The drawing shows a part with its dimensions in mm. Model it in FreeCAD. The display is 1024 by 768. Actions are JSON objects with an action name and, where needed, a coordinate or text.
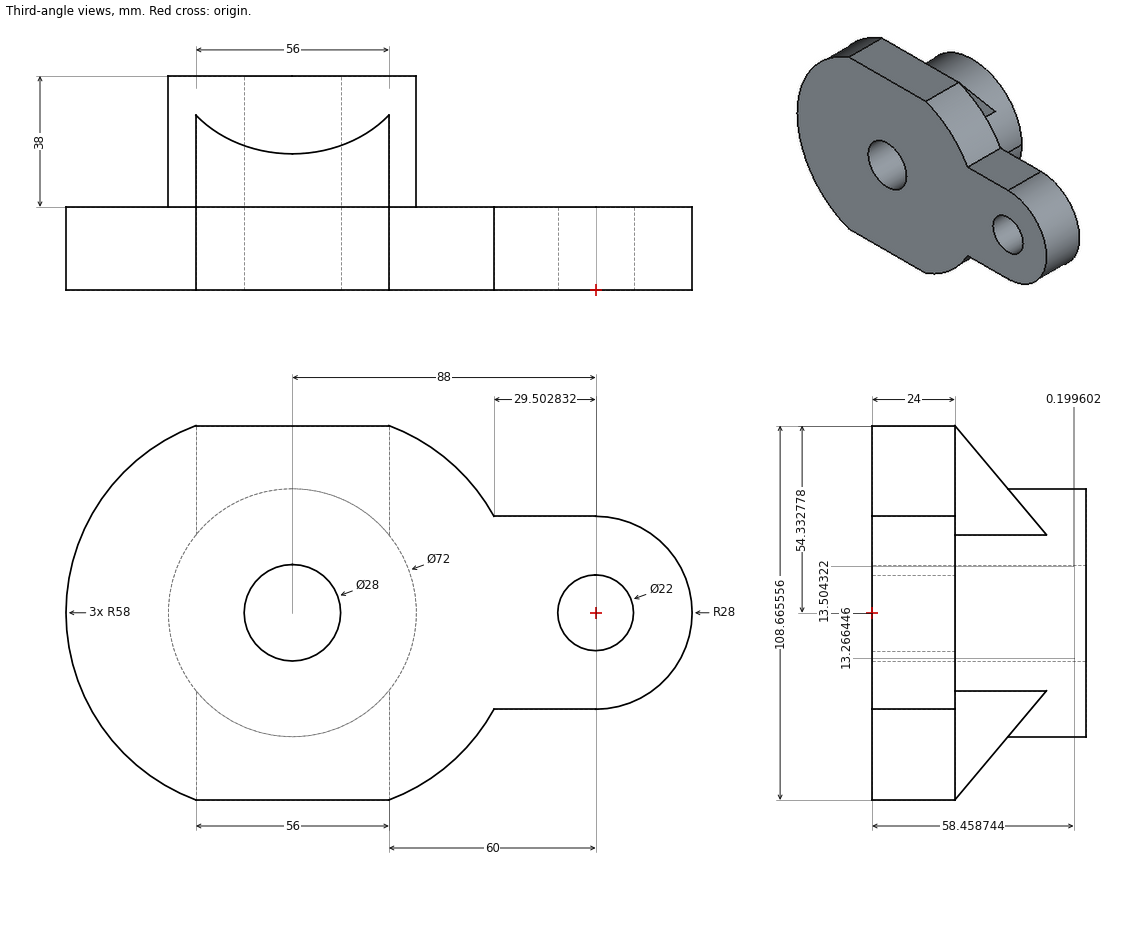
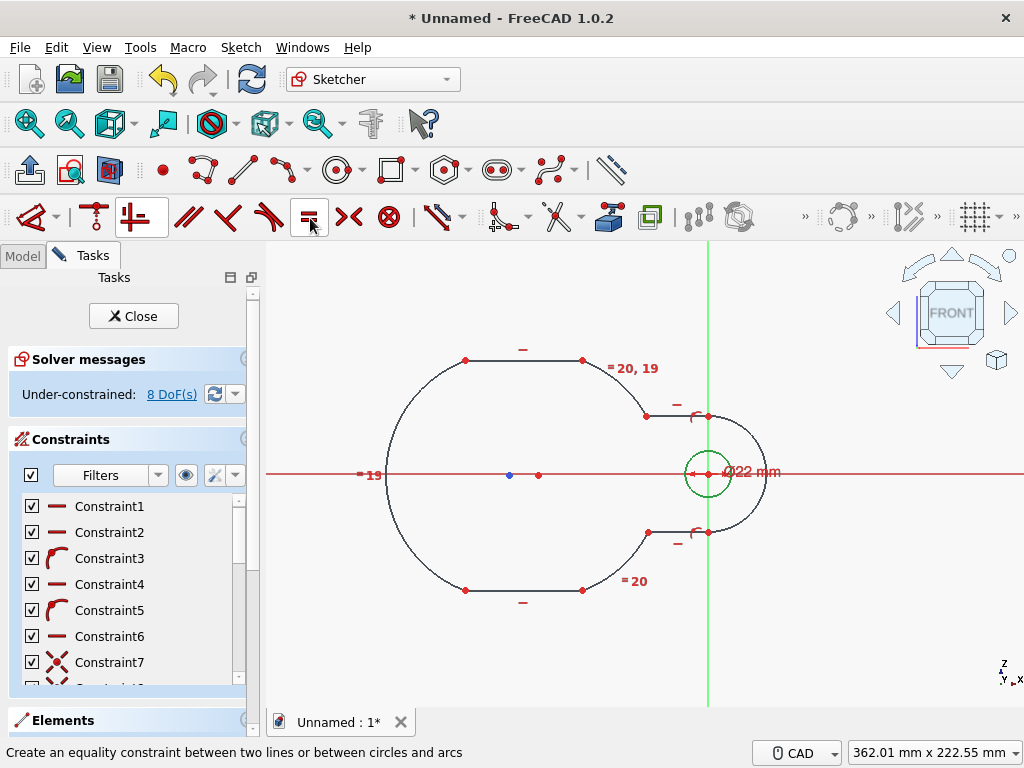
{"action": "left_click", "coordinate": [509, 476]}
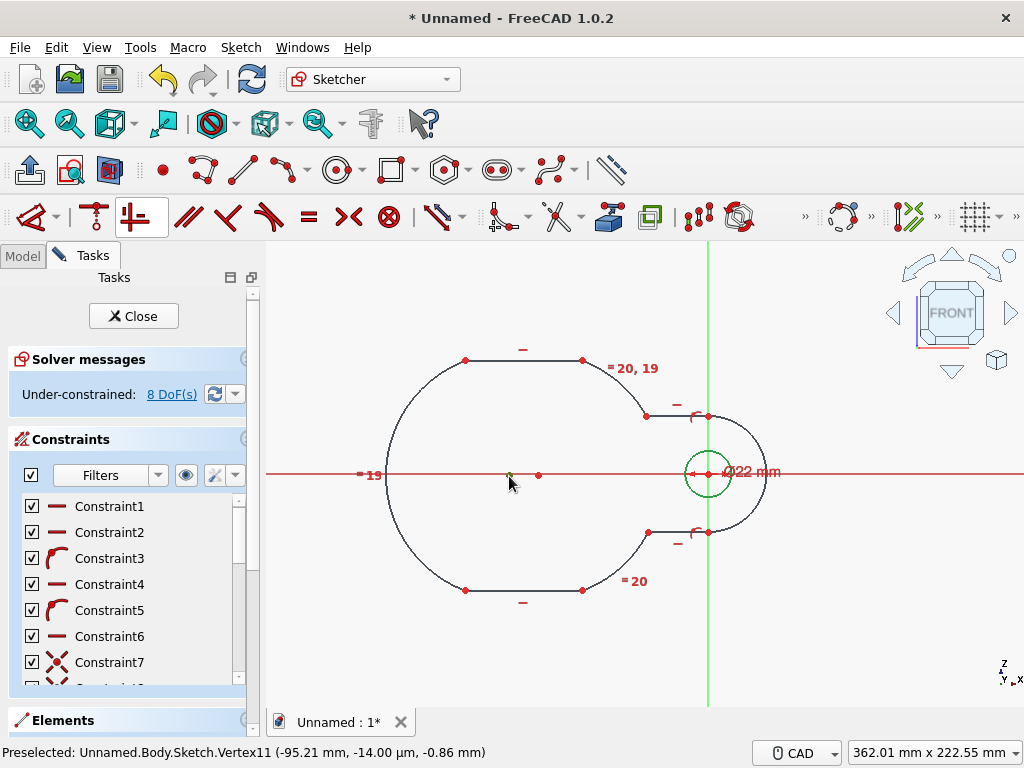
{"action": "left_click", "coordinate": [334, 474]}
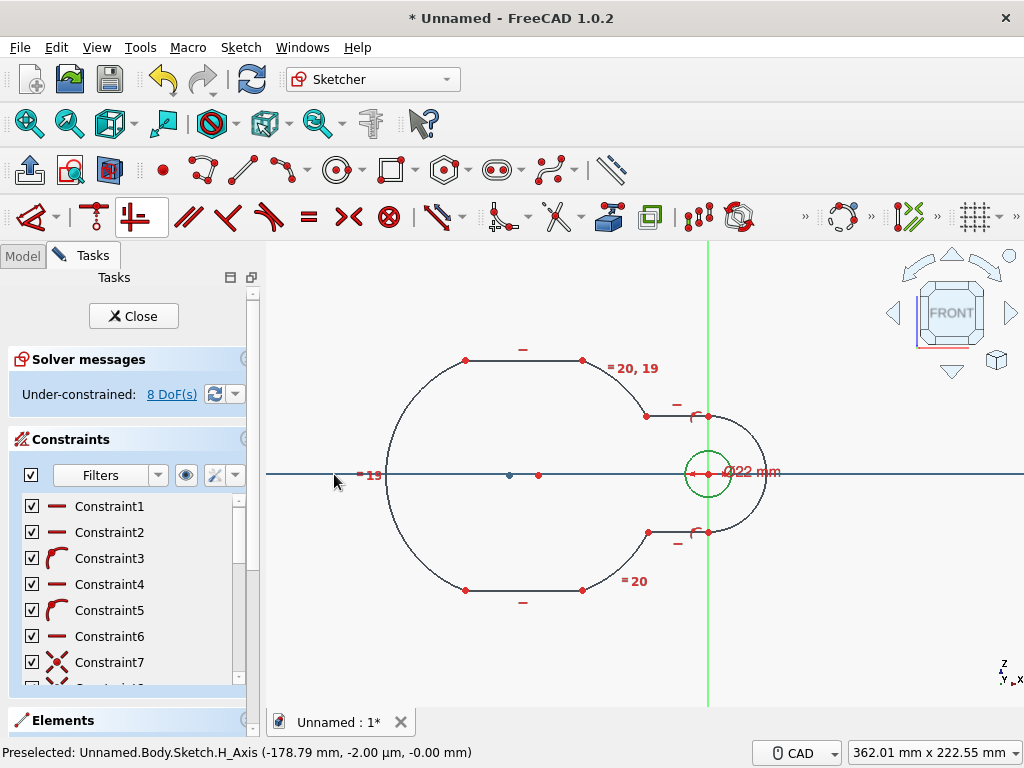
{"action": "left_click", "coordinate": [94, 218]}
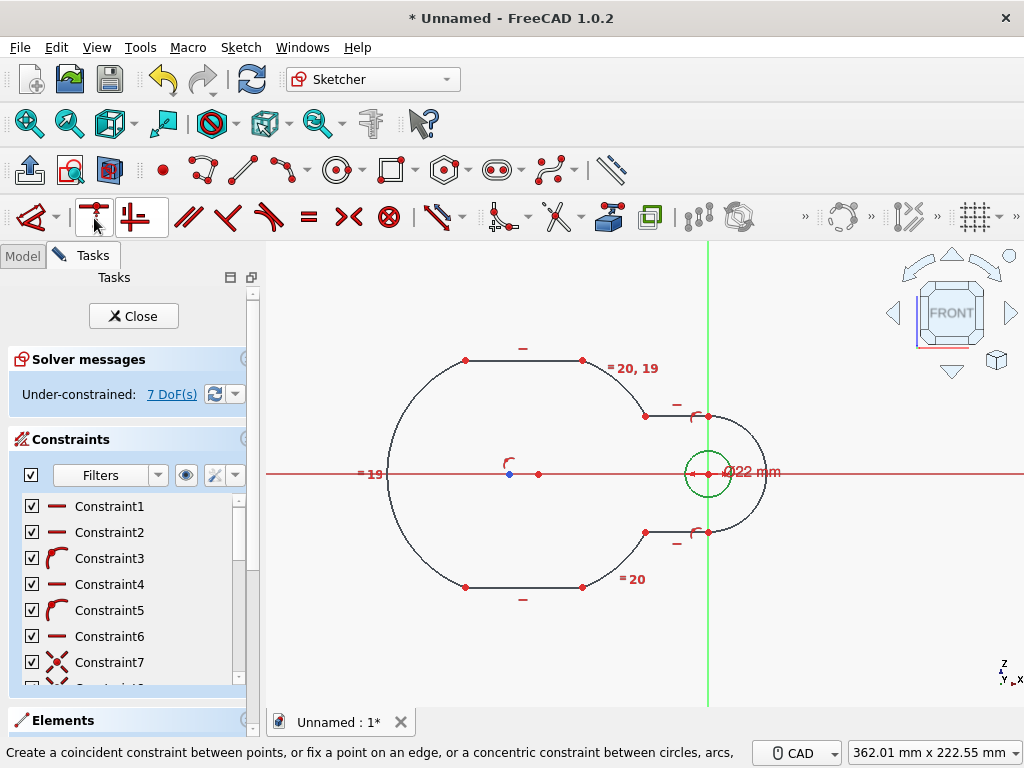
{"action": "left_click", "coordinate": [539, 474]}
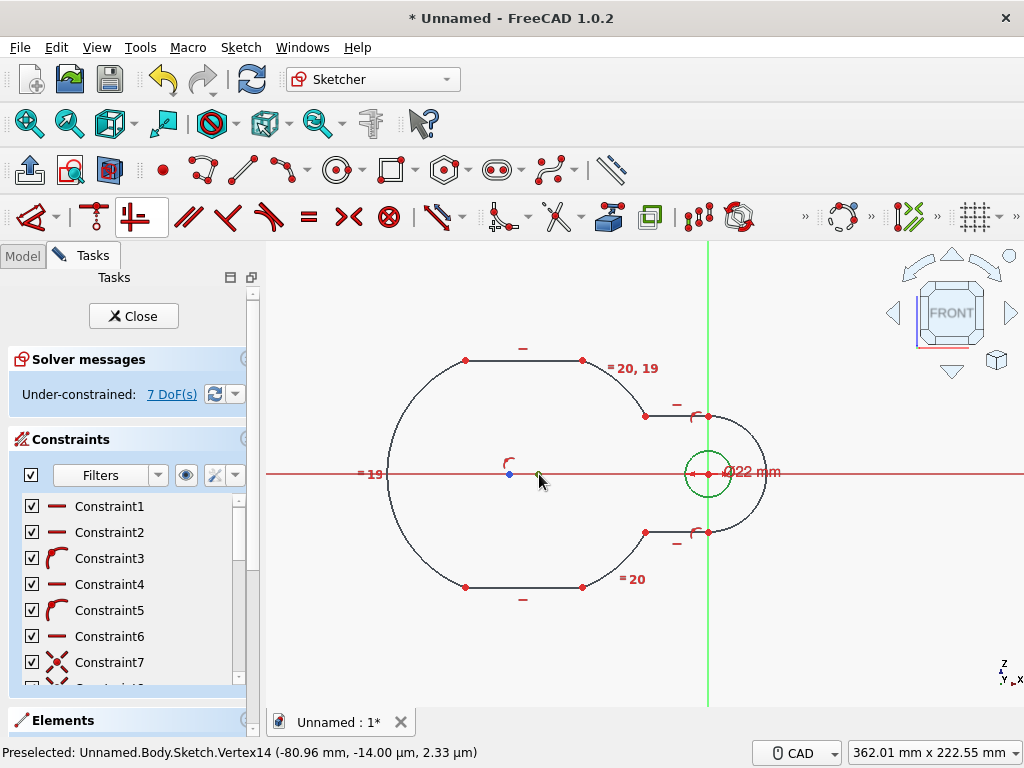
{"action": "left_click", "coordinate": [334, 474]}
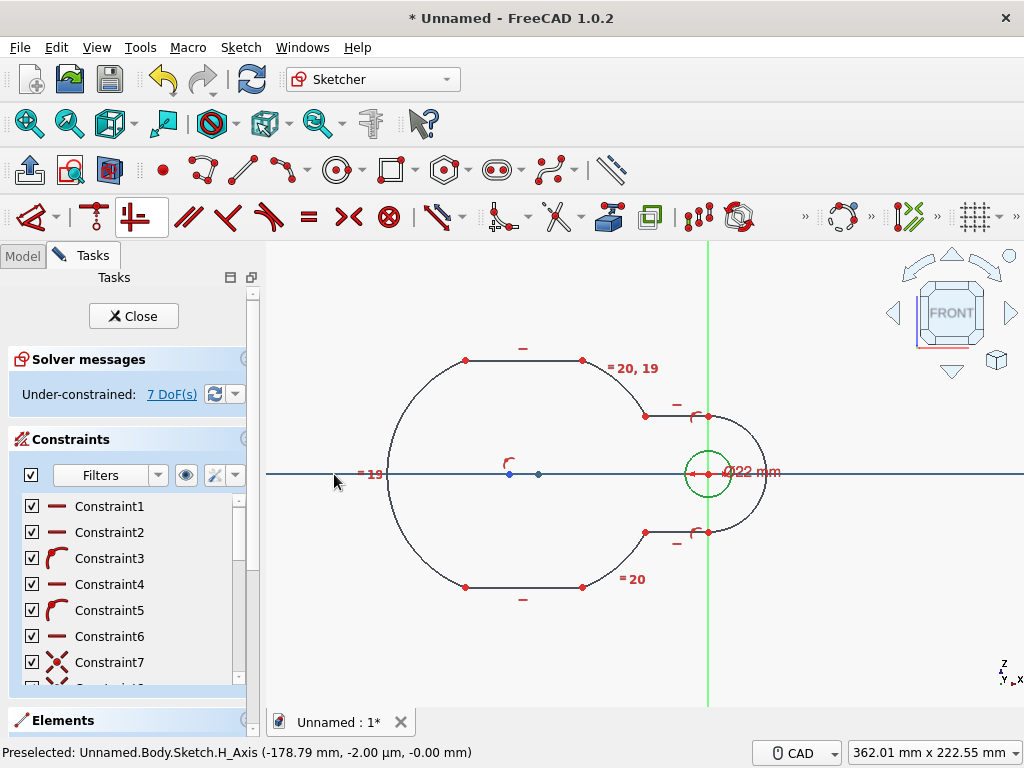
{"action": "key", "text": "c"}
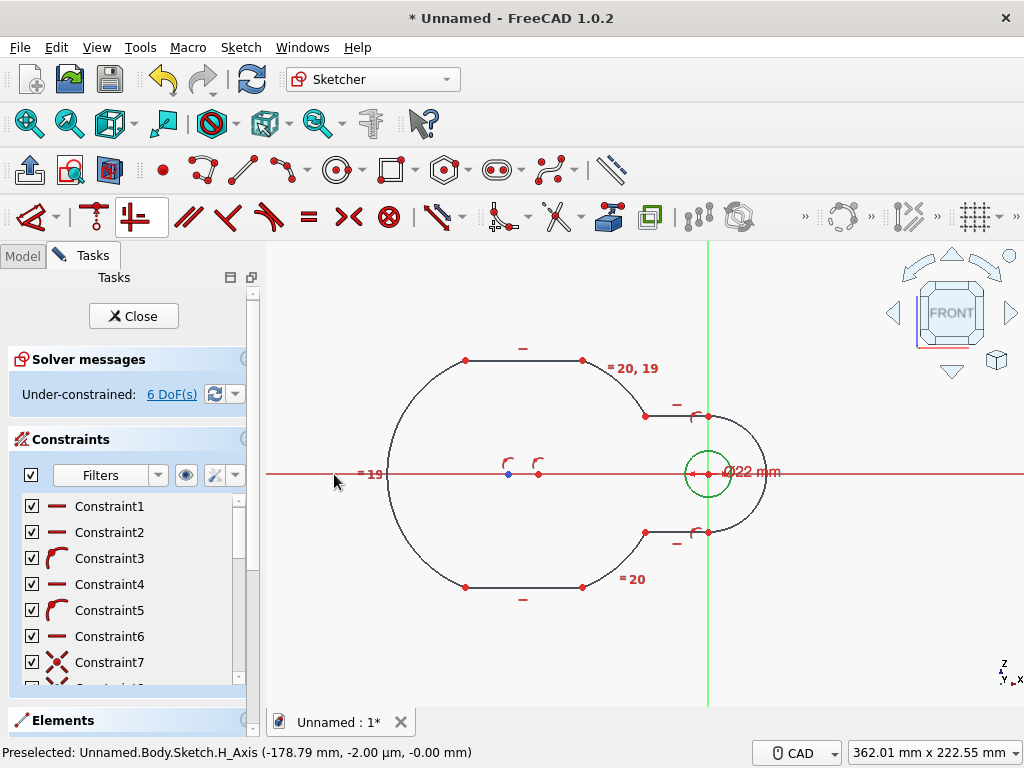
{"action": "left_click", "coordinate": [32, 218]}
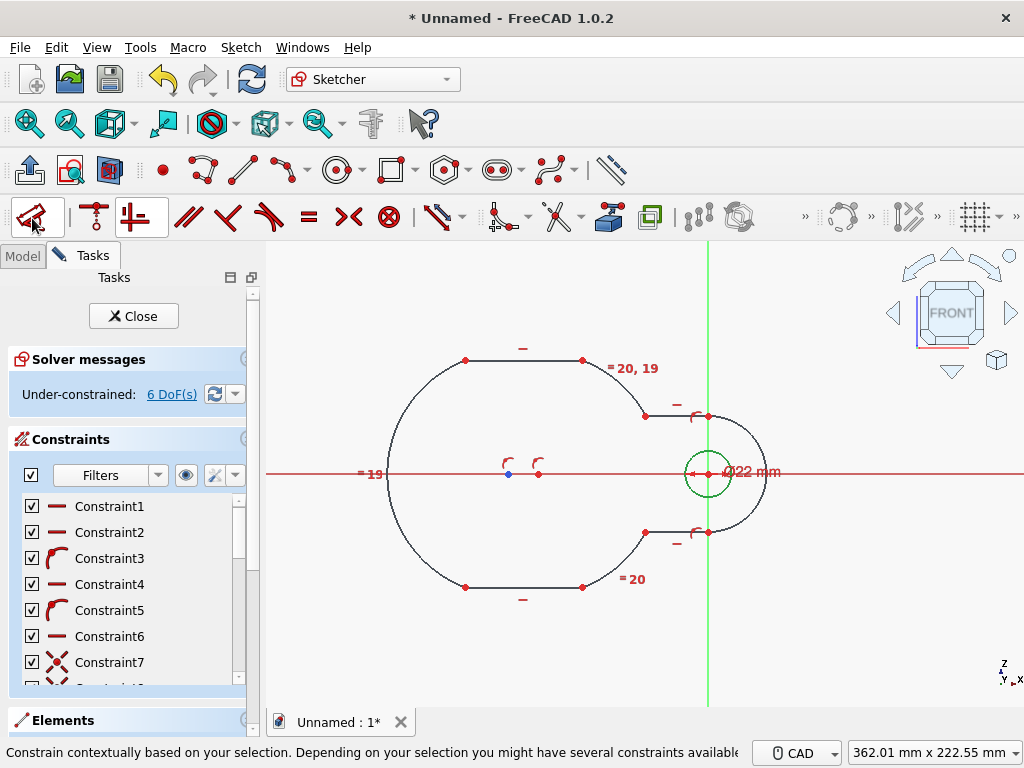
{"action": "left_click", "coordinate": [401, 418]}
{"action": "left_click", "coordinate": [373, 403]}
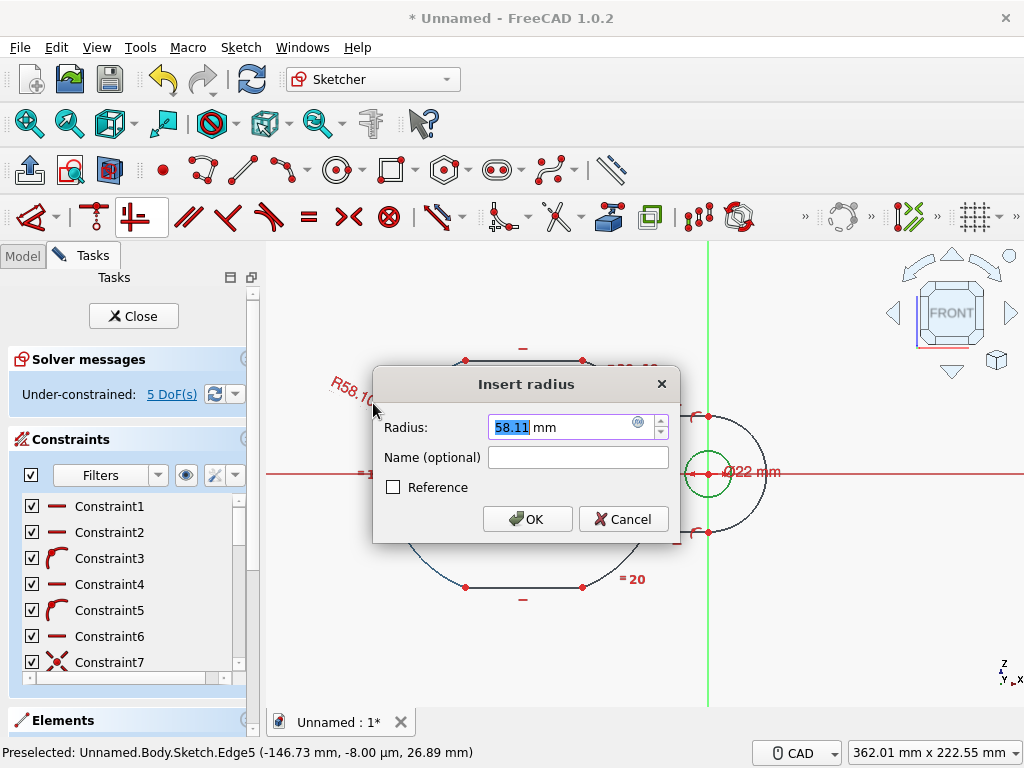
{"action": "type", "text": "58"}
{"action": "key", "text": "Return"}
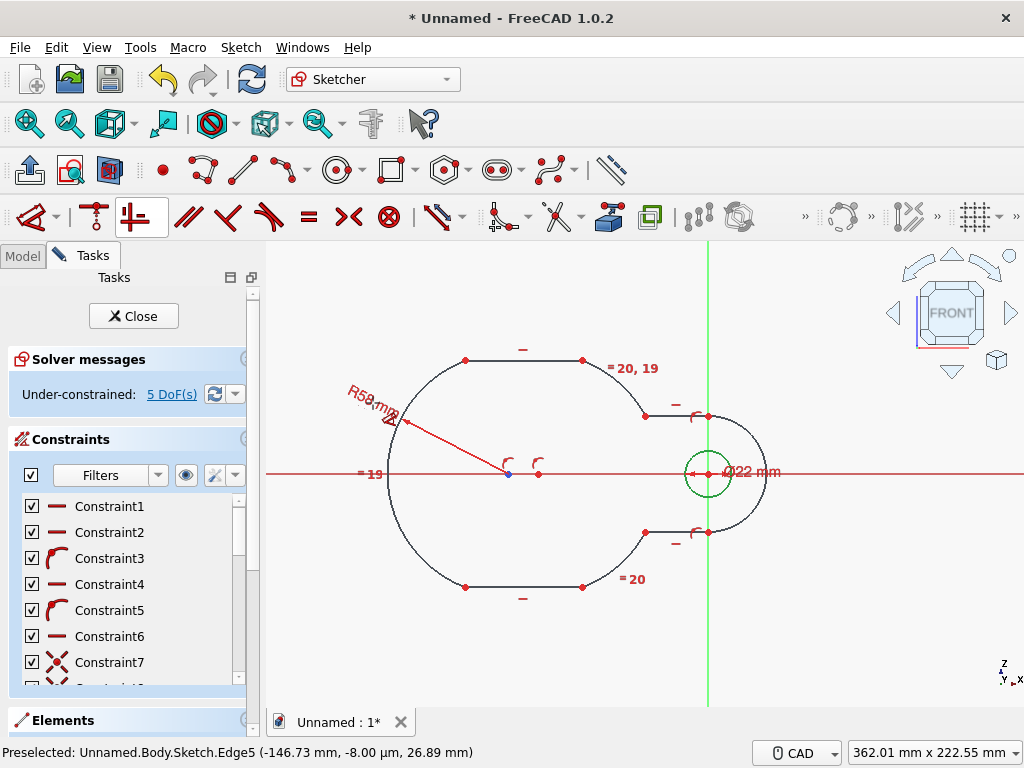
{"action": "left_click", "coordinate": [755, 508]}
{"action": "left_click", "coordinate": [781, 527]}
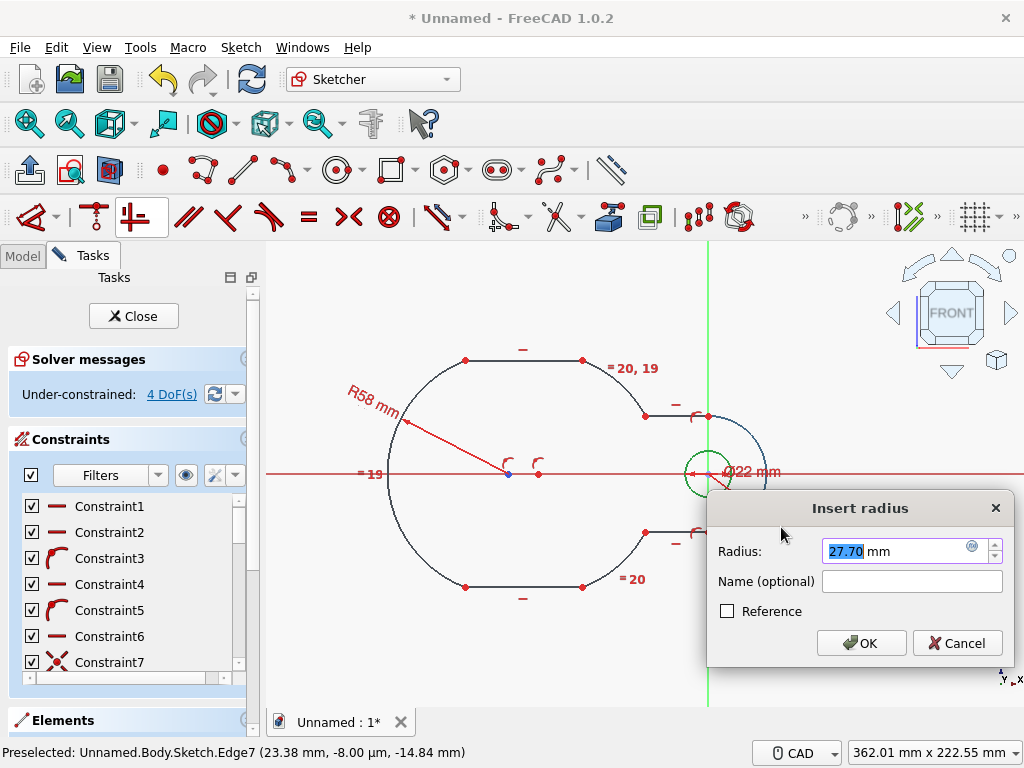
{"action": "type", "text": "28"}
{"action": "key", "text": "Return"}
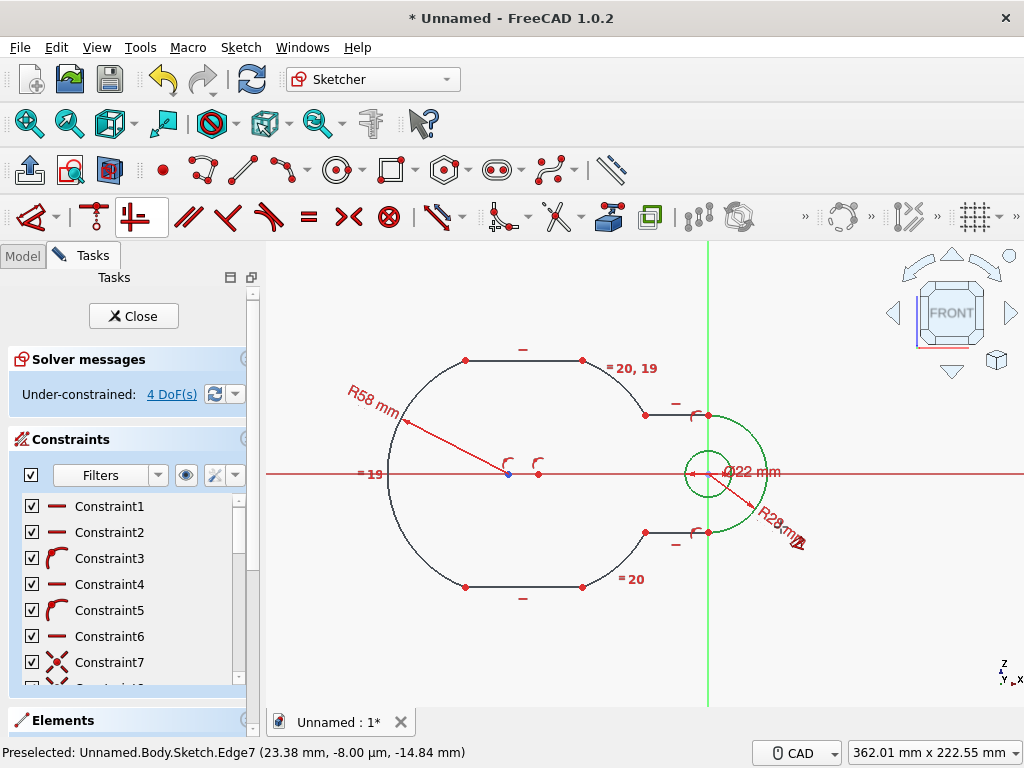
{"action": "left_click", "coordinate": [547, 587]}
{"action": "left_click", "coordinate": [524, 621]}